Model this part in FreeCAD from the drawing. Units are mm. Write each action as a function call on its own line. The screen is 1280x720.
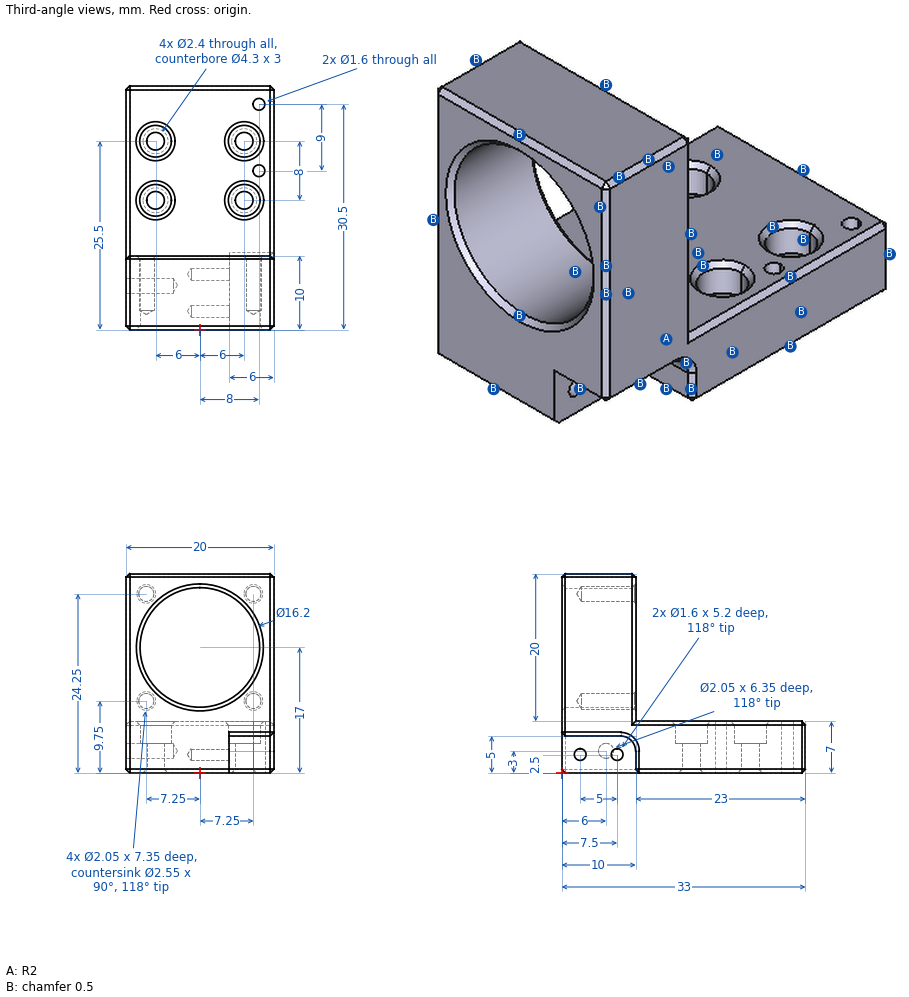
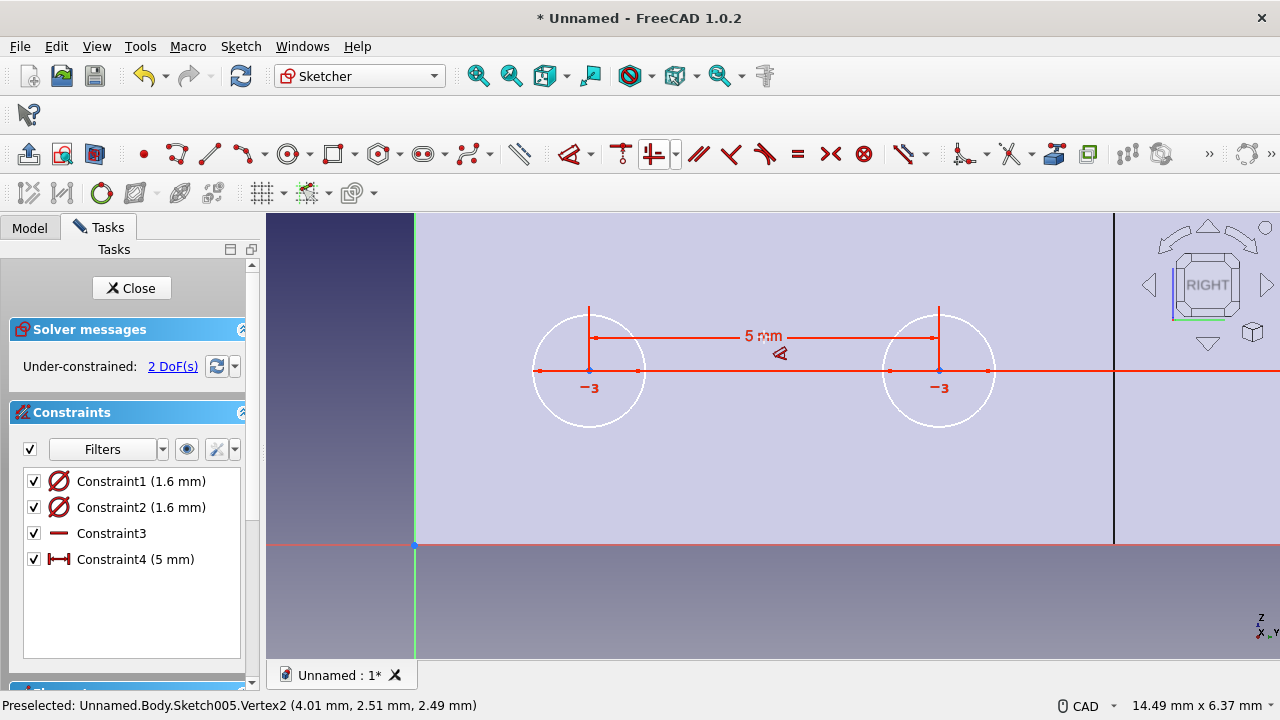
click(939, 371)
click(677, 579)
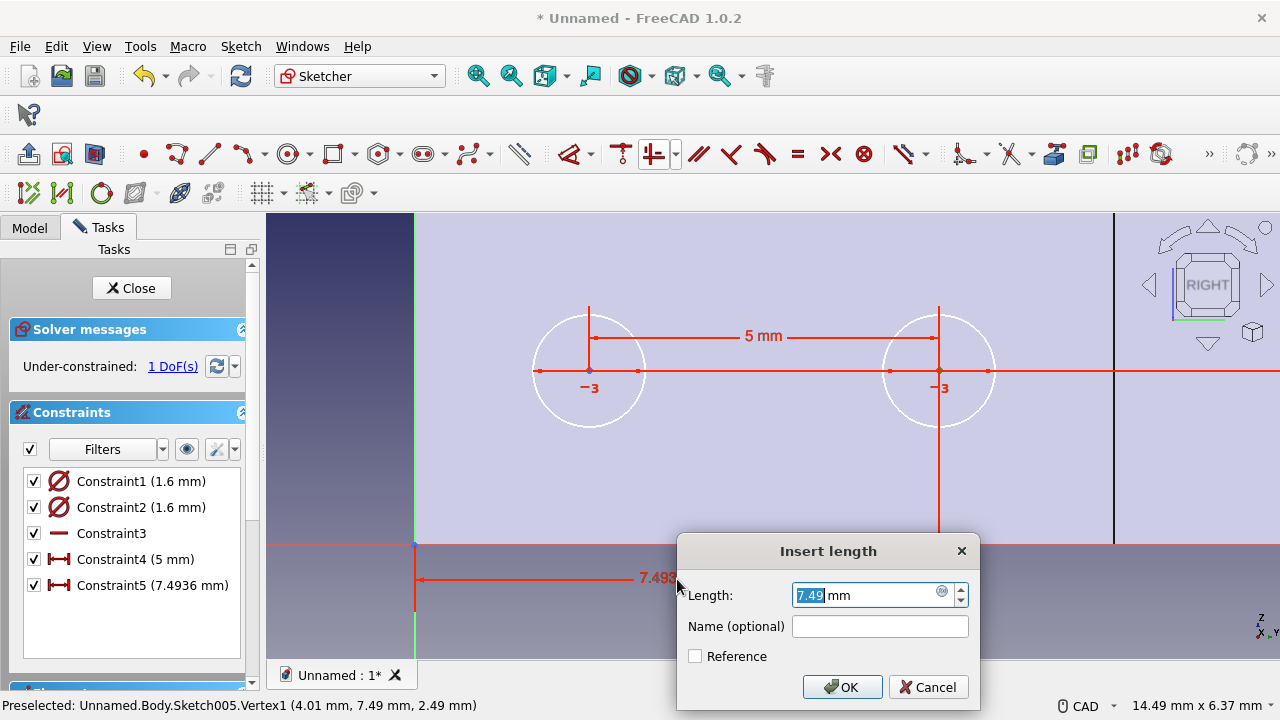
text(7.5)
key(Return)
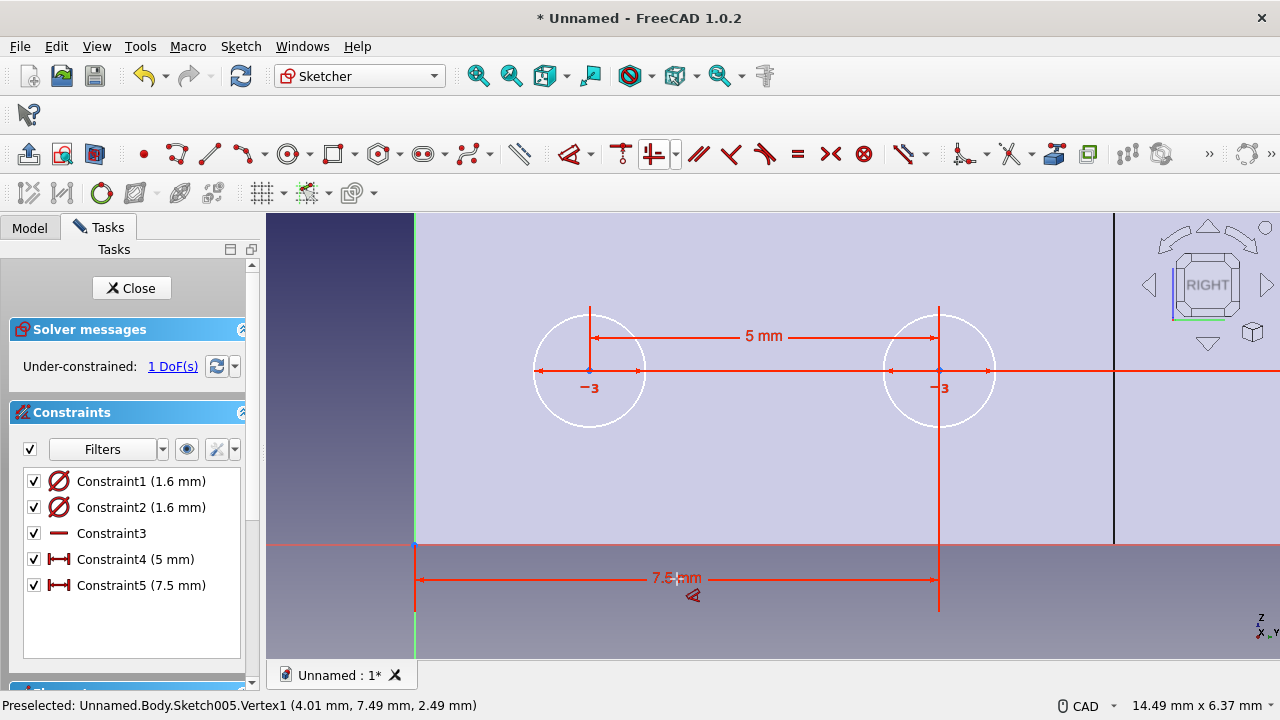
click(939, 371)
click(381, 458)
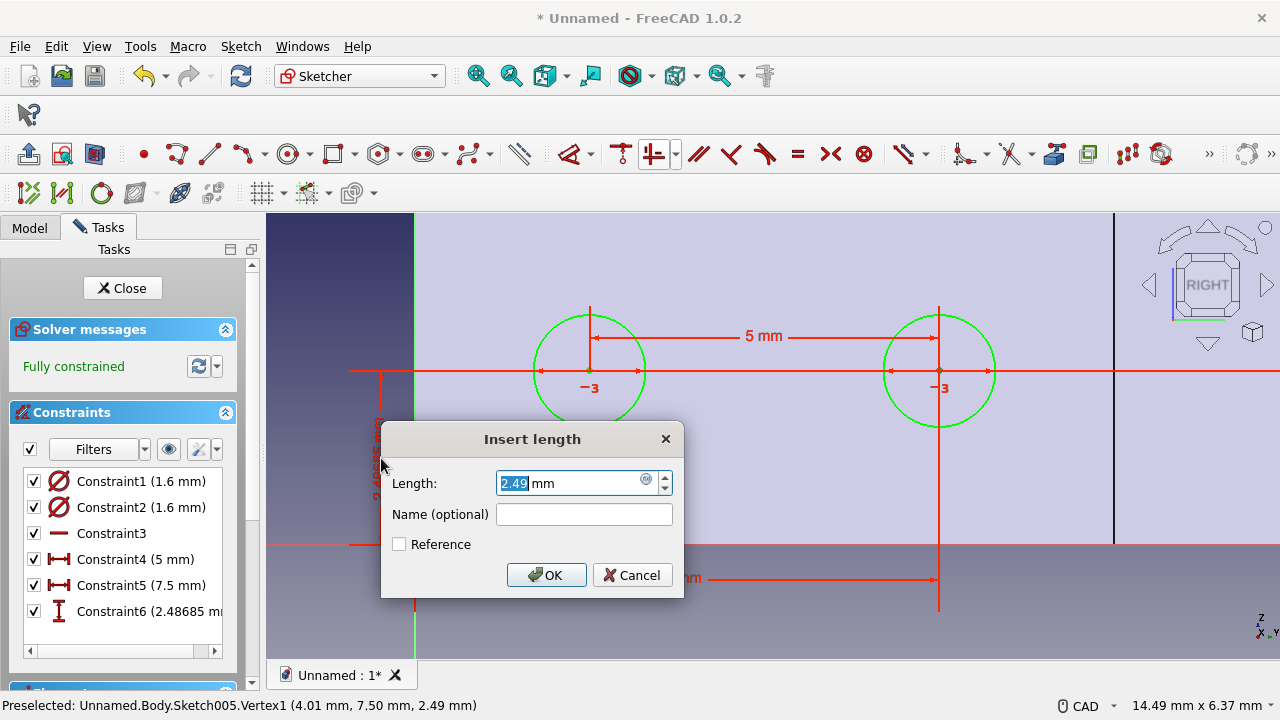
text(2.5)
key(Return)
key(Escape)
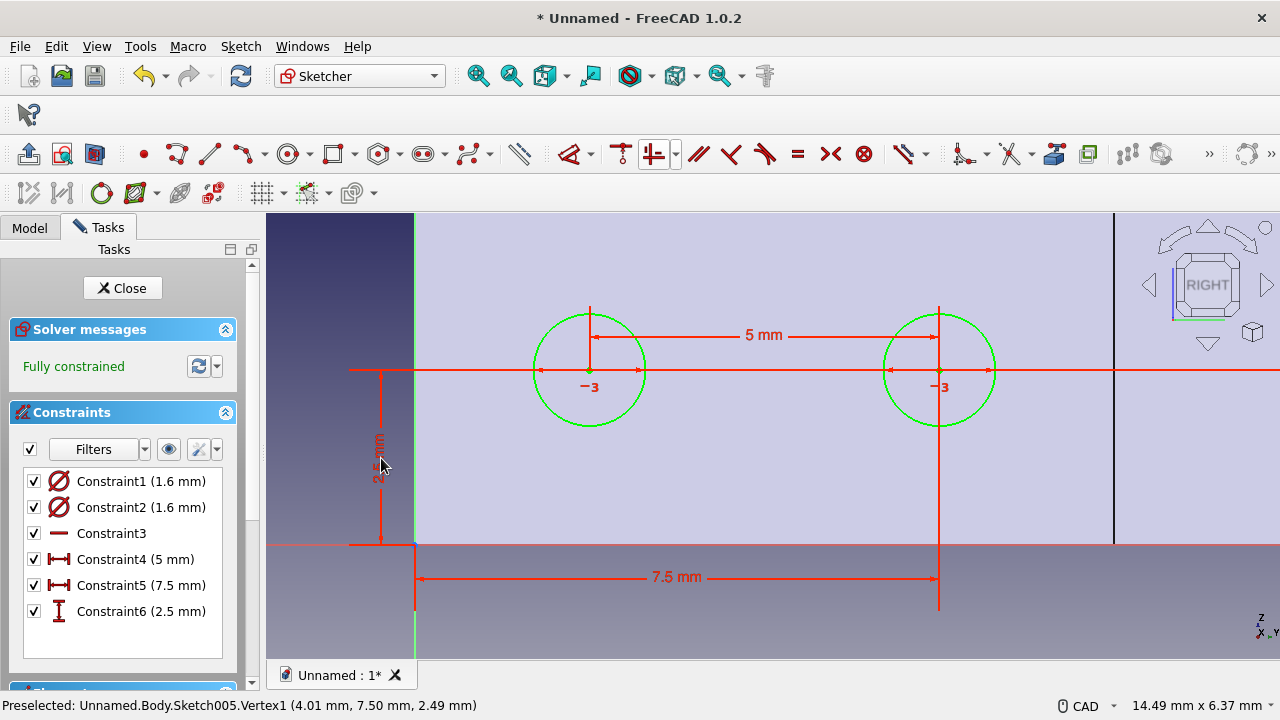
click(123, 288)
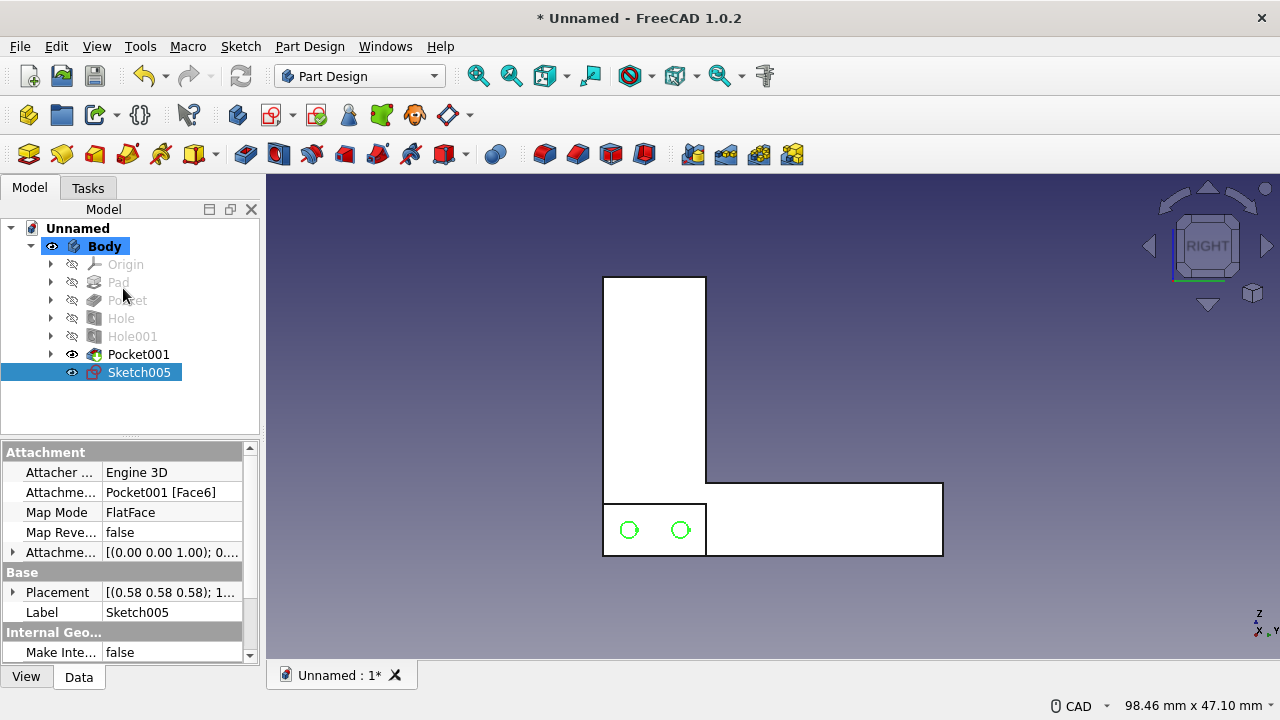
click(279, 154)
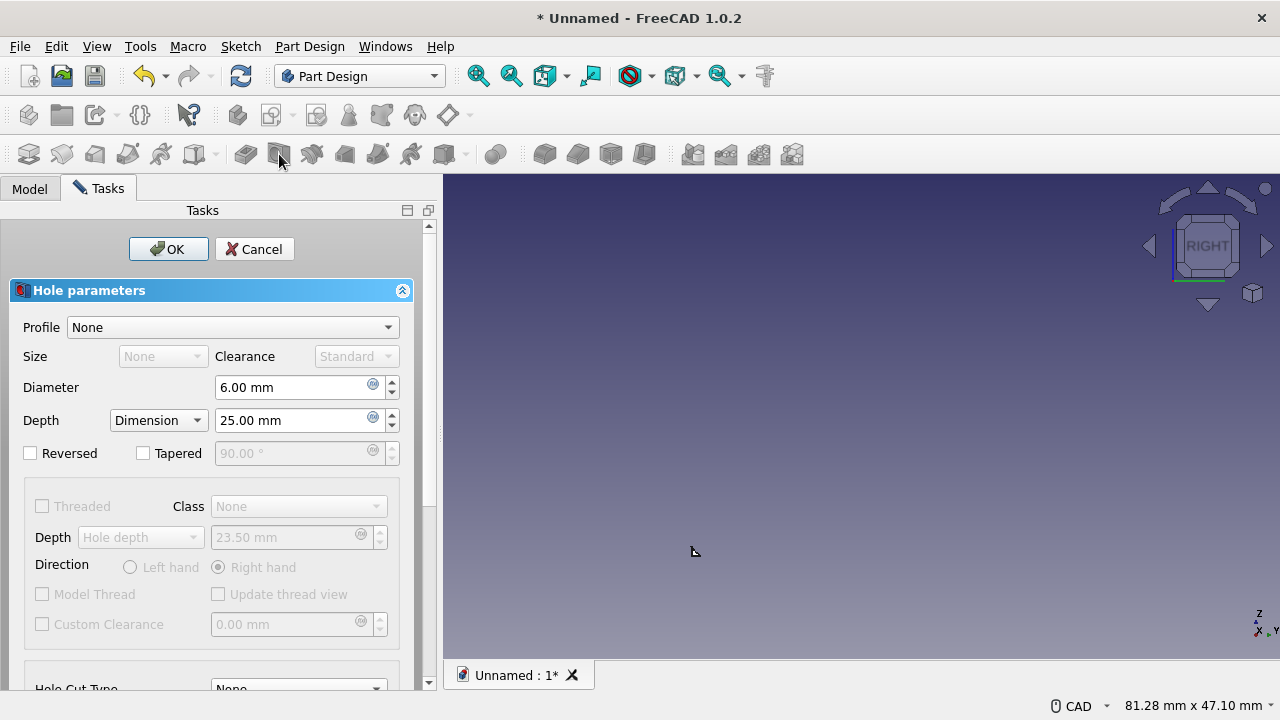
triple_click(300, 388)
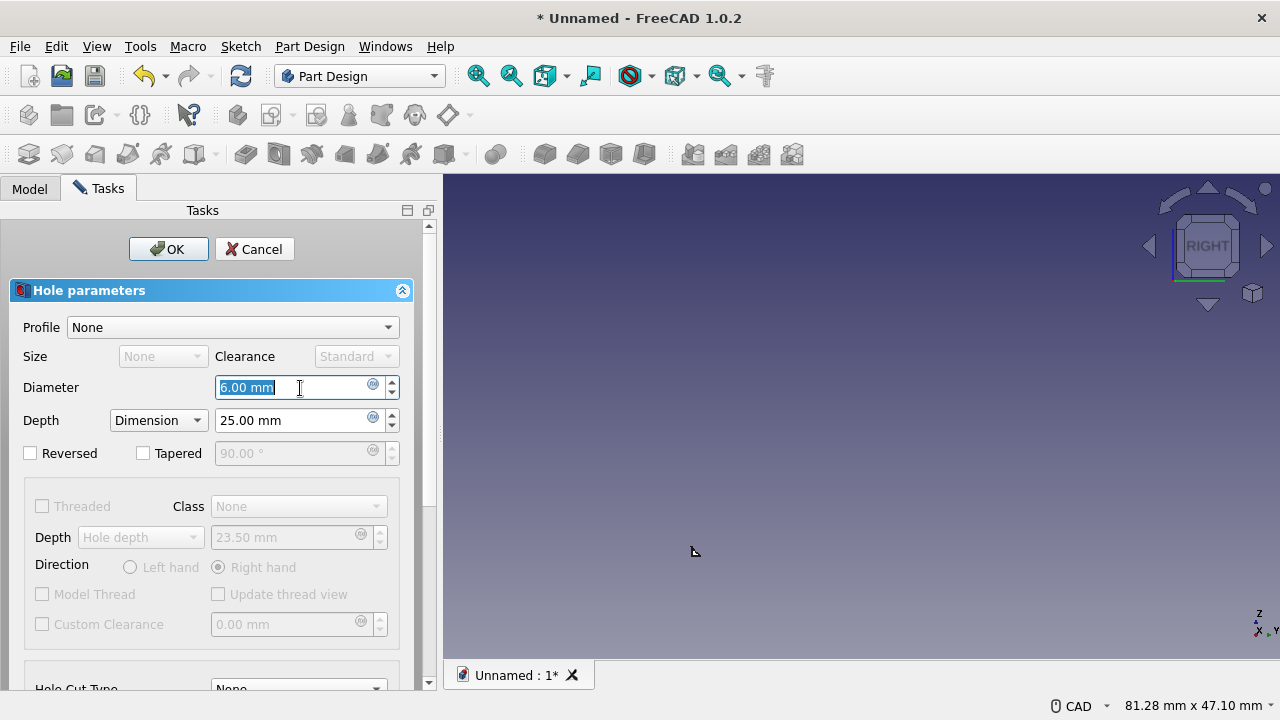
text(1.6)
key(Tab)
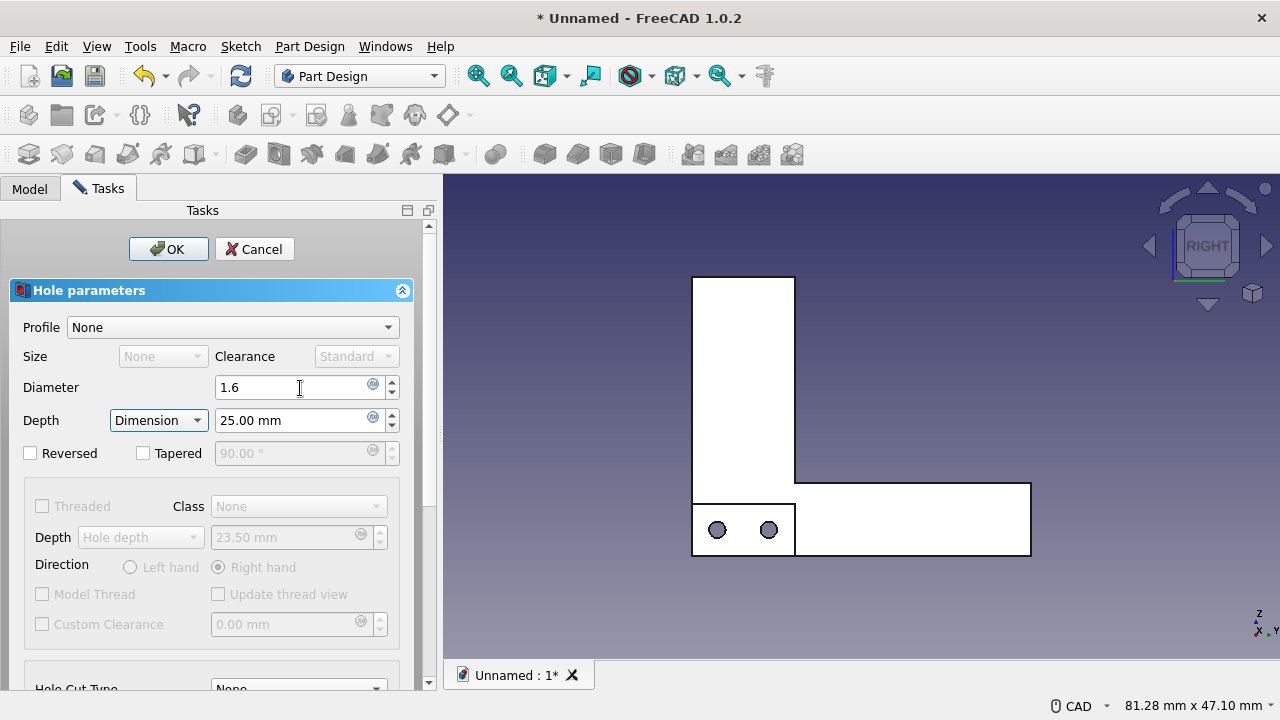
triple_click(300, 420)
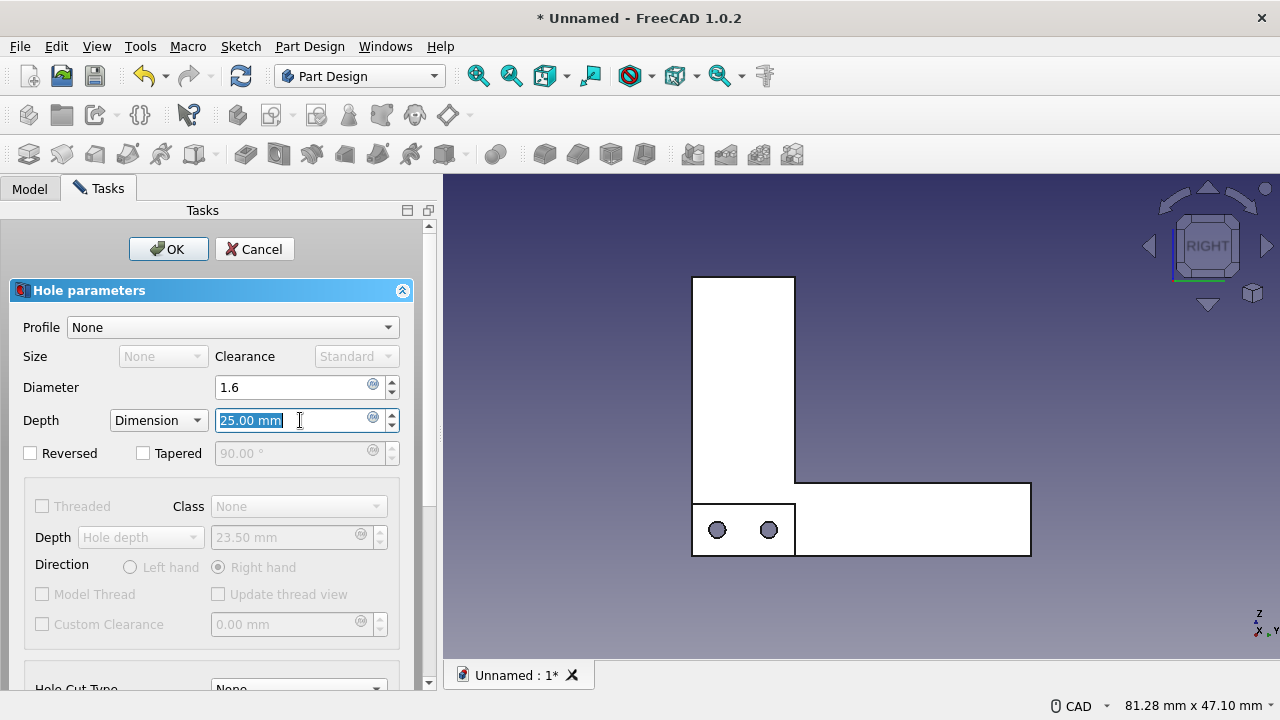
text(5.2)
key(Tab)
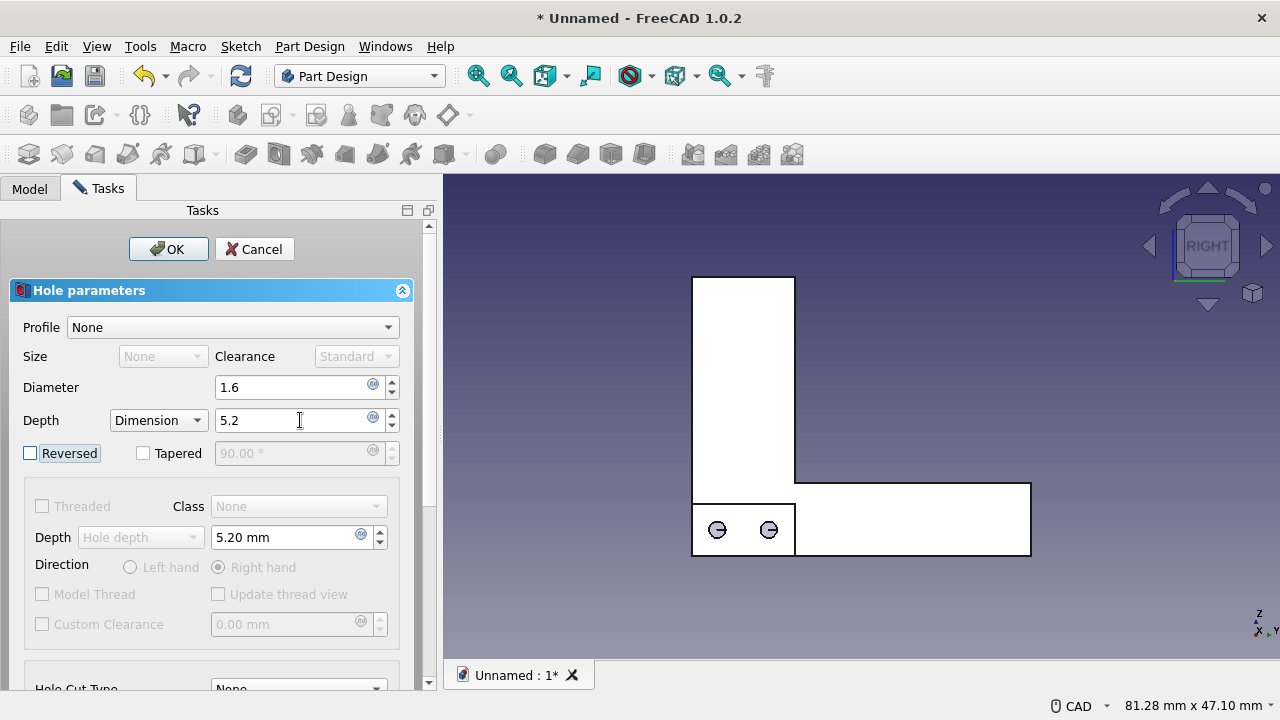
click(169, 249)